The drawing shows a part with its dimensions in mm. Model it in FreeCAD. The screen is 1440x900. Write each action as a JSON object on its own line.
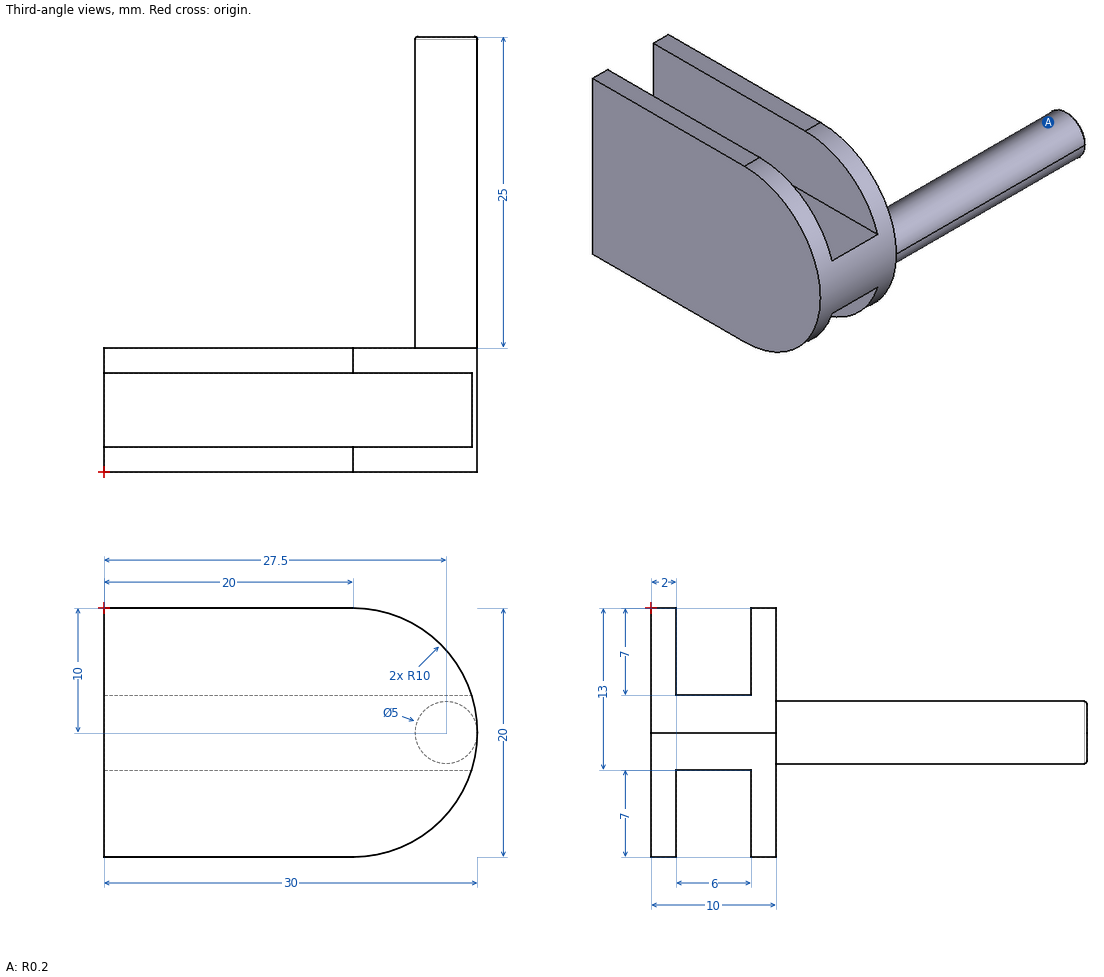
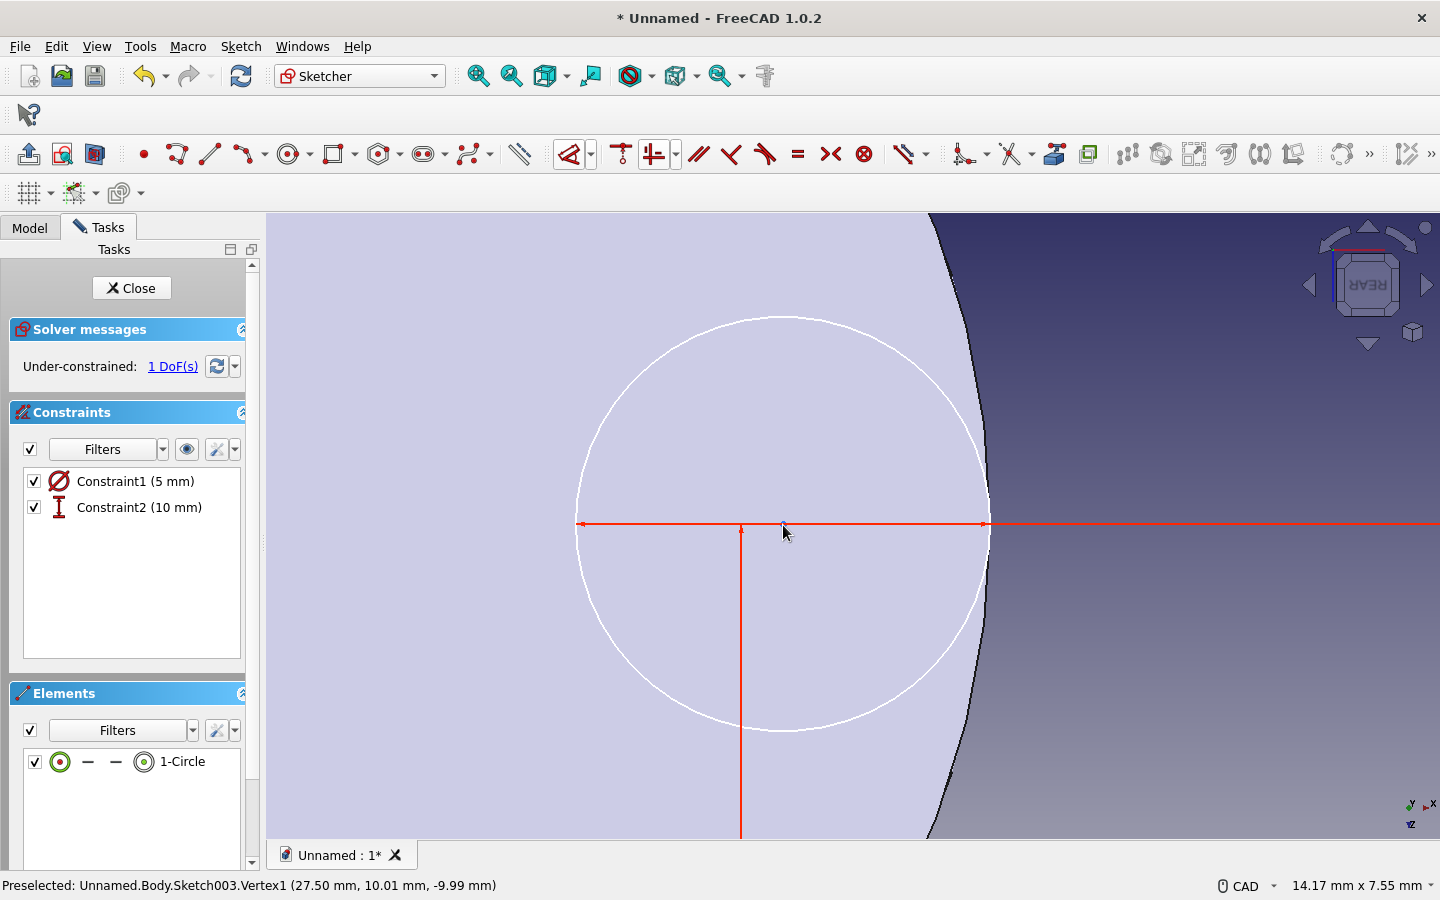
{"action": "left_click", "coordinate": [783, 524]}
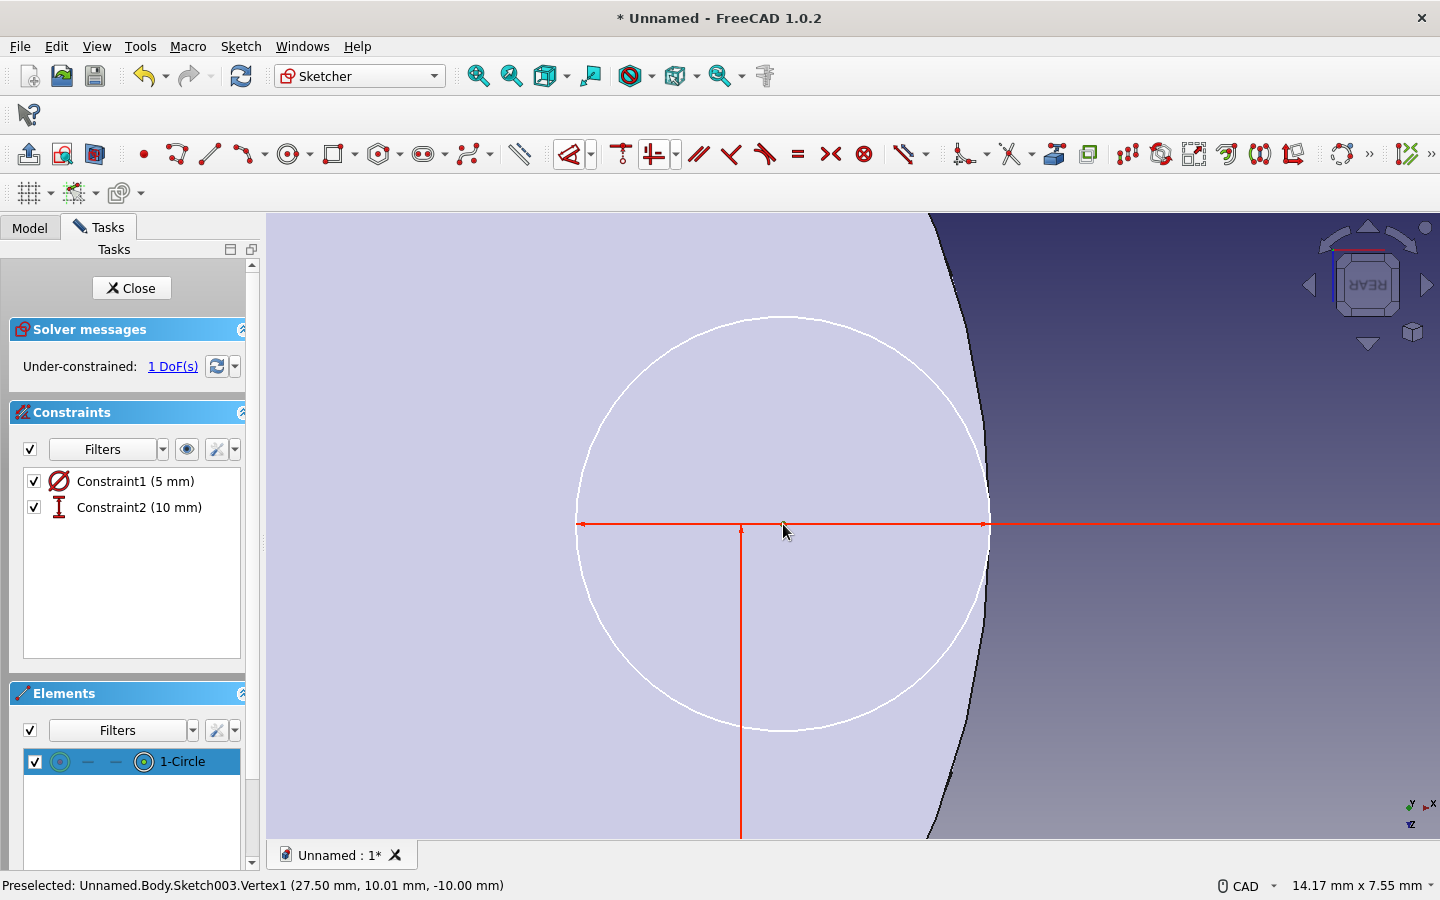
{"action": "key", "text": "l"}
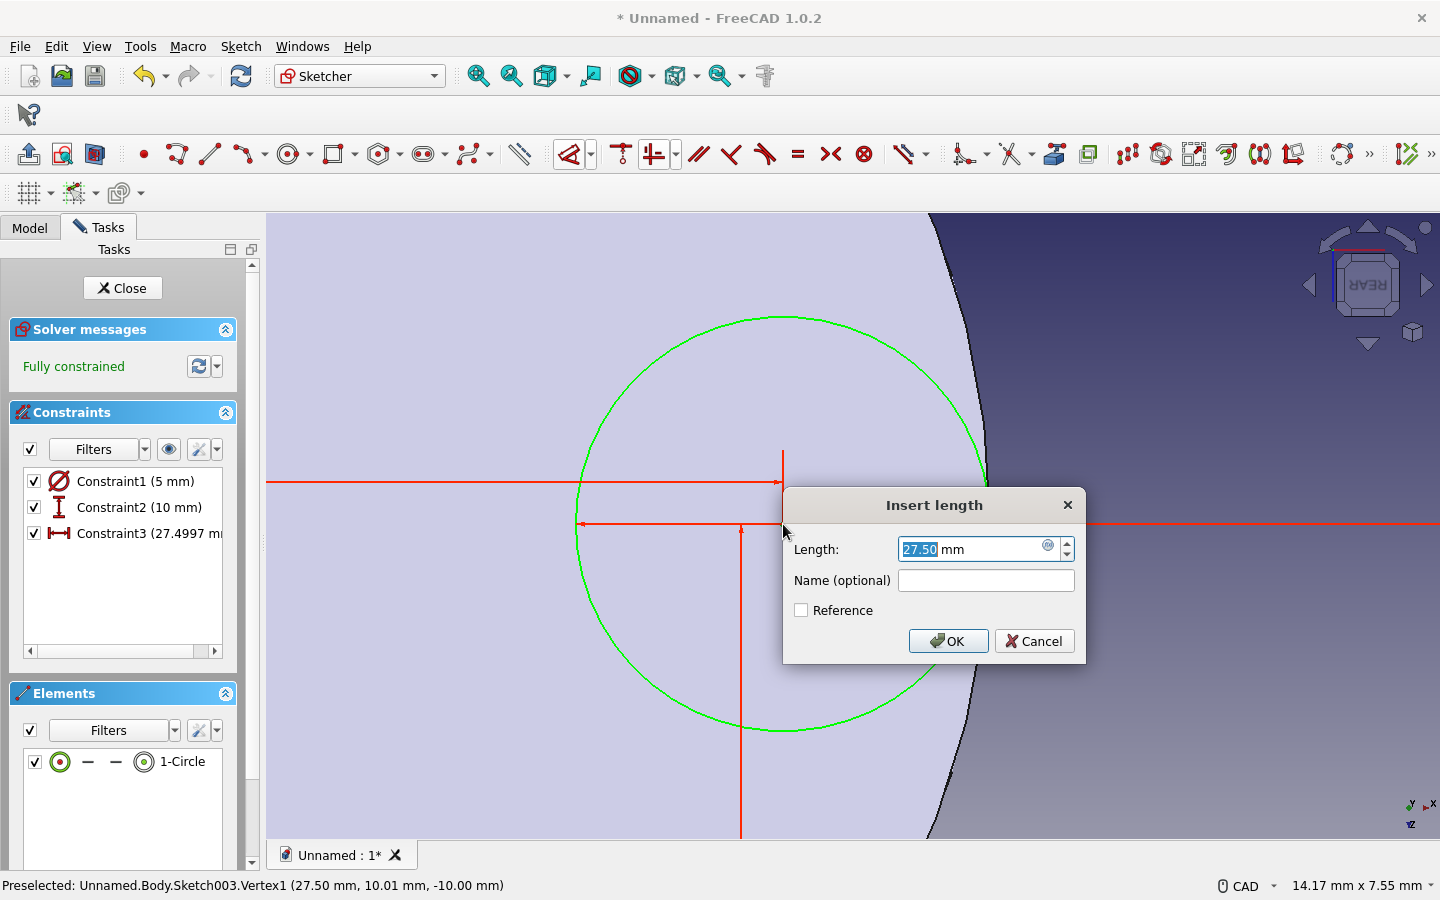
{"action": "type", "text": "27.5"}
{"action": "key", "text": "Return"}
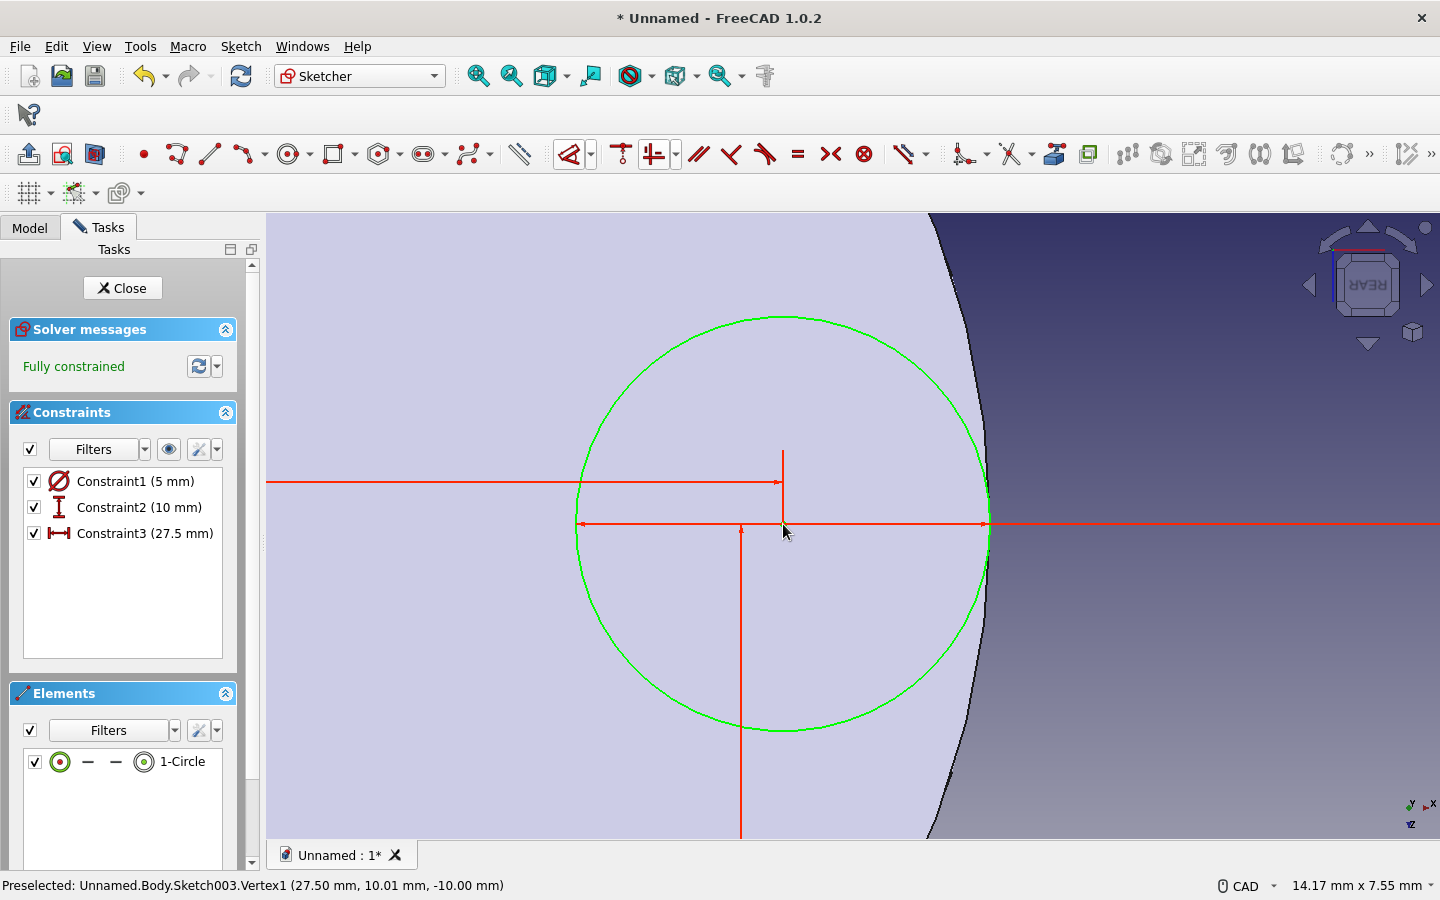
{"action": "left_click", "coordinate": [123, 288]}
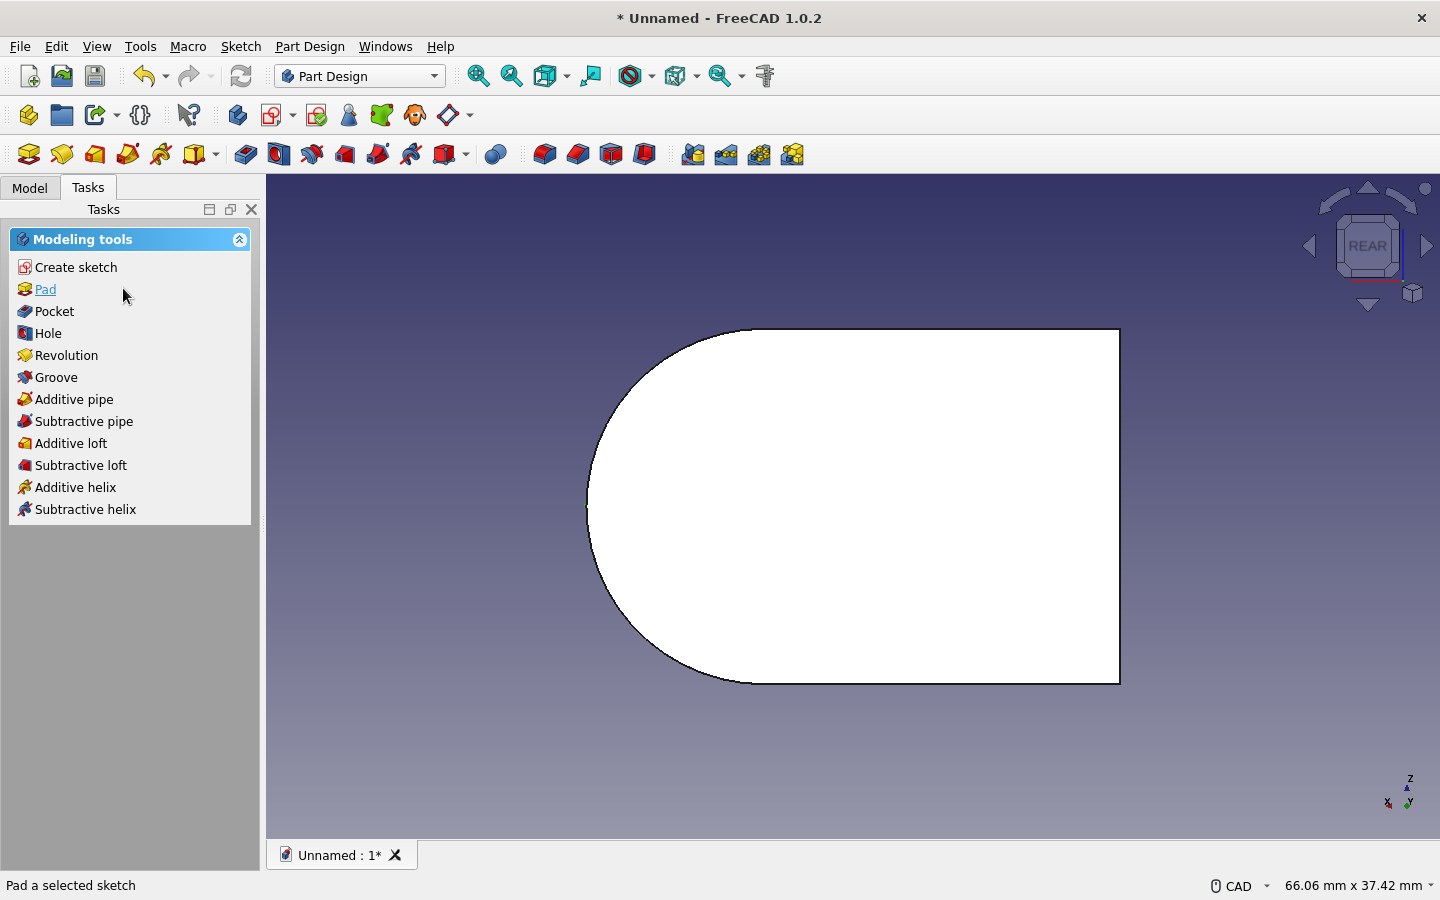
{"action": "left_click", "coordinate": [29, 154]}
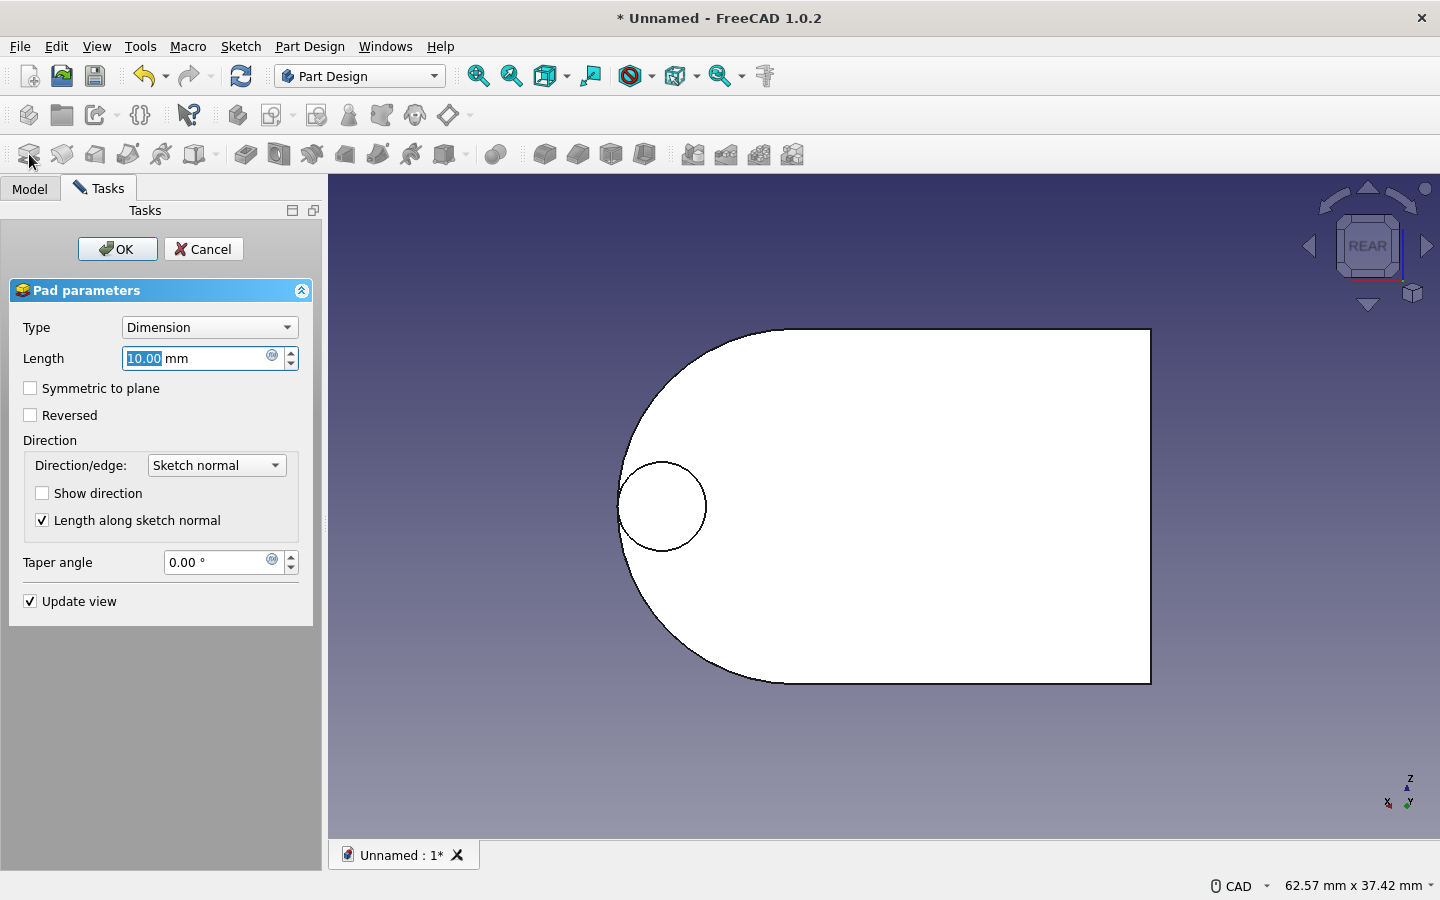
{"action": "type", "text": "25"}
{"action": "key", "text": "Tab"}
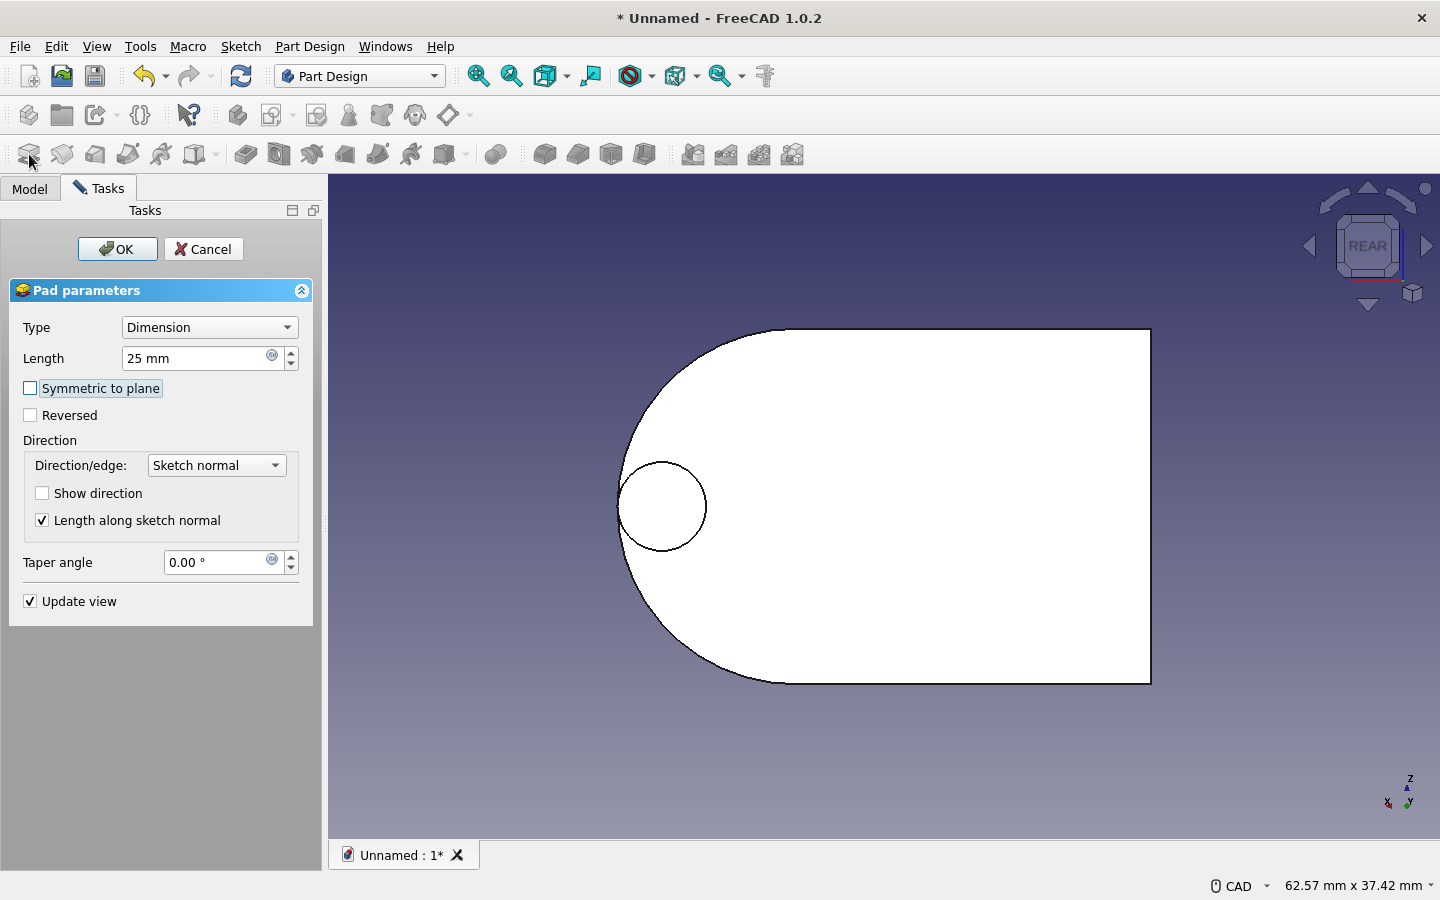
{"action": "left_click", "coordinate": [118, 249]}